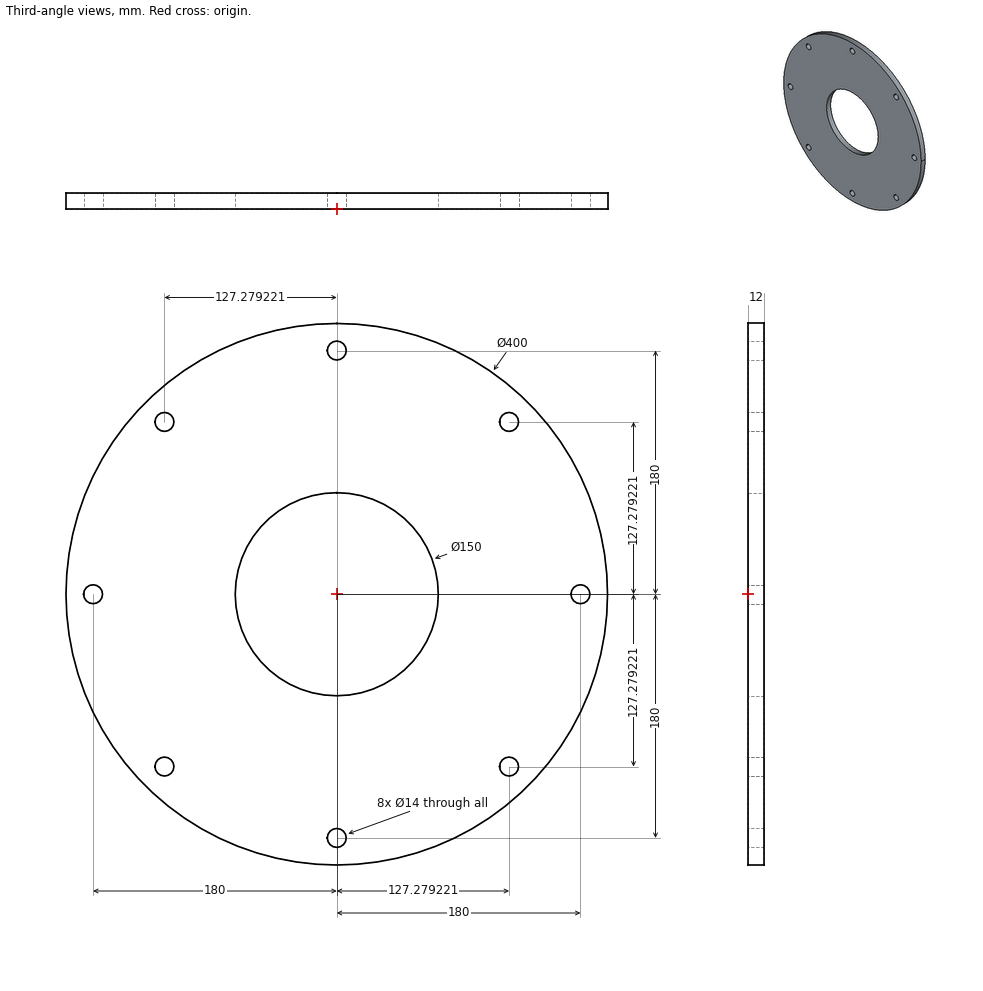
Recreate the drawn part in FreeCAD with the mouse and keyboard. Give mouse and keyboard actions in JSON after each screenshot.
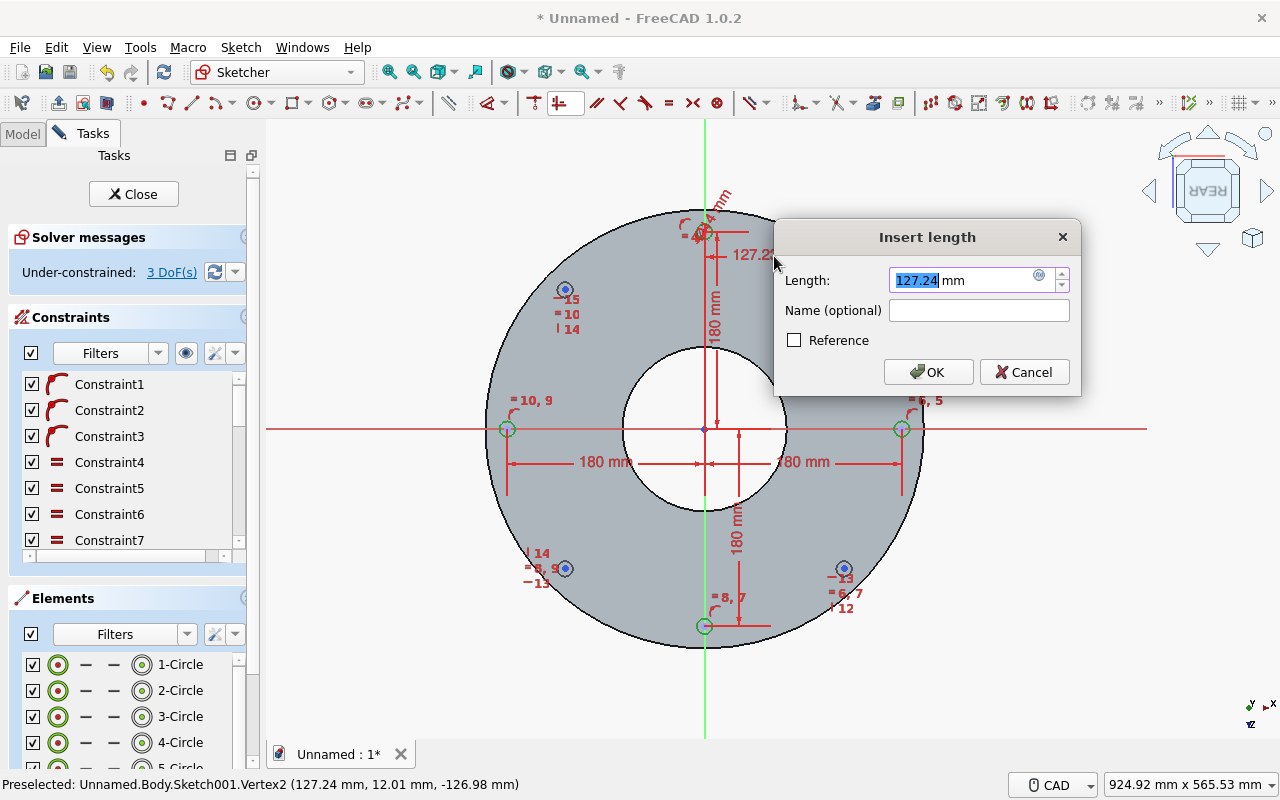
{"action": "type", "text": "127.279221"}
{"action": "key", "text": "Return"}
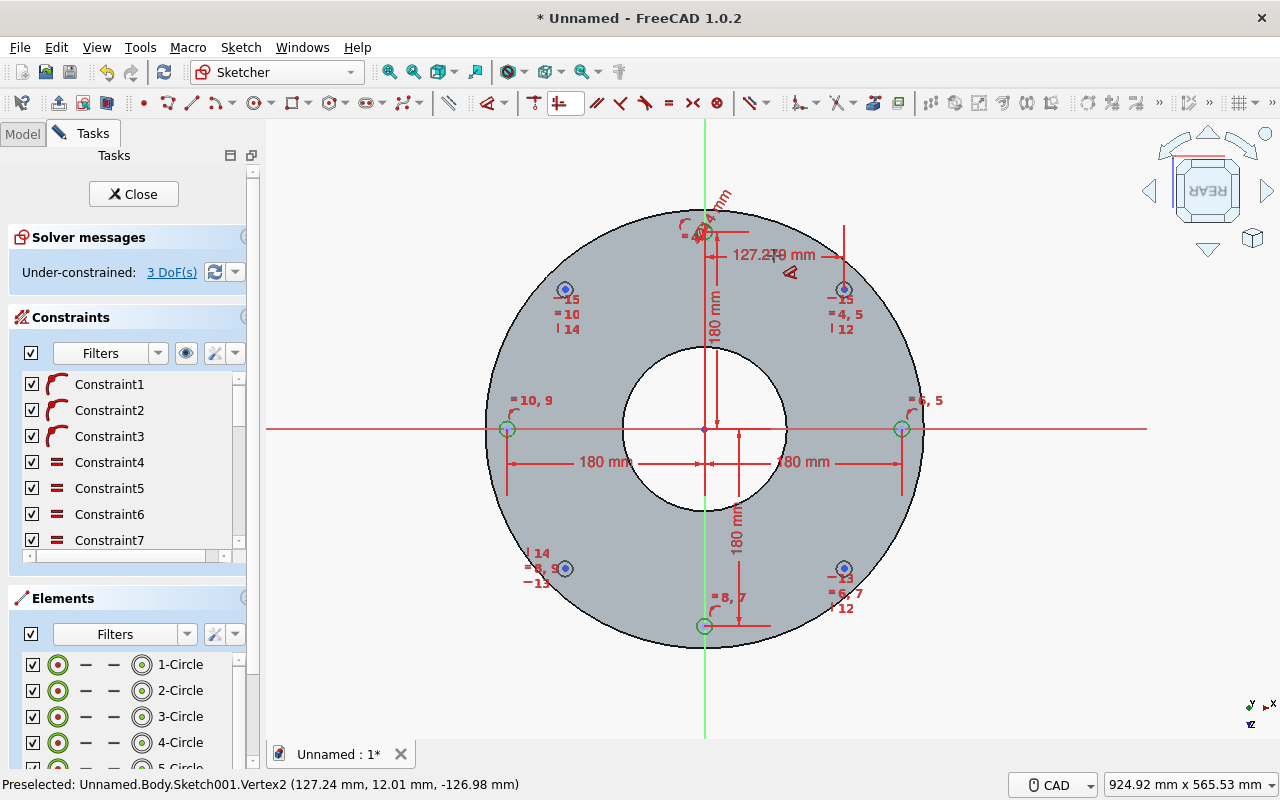
{"action": "left_click", "coordinate": [844, 290]}
{"action": "left_click", "coordinate": [878, 360]}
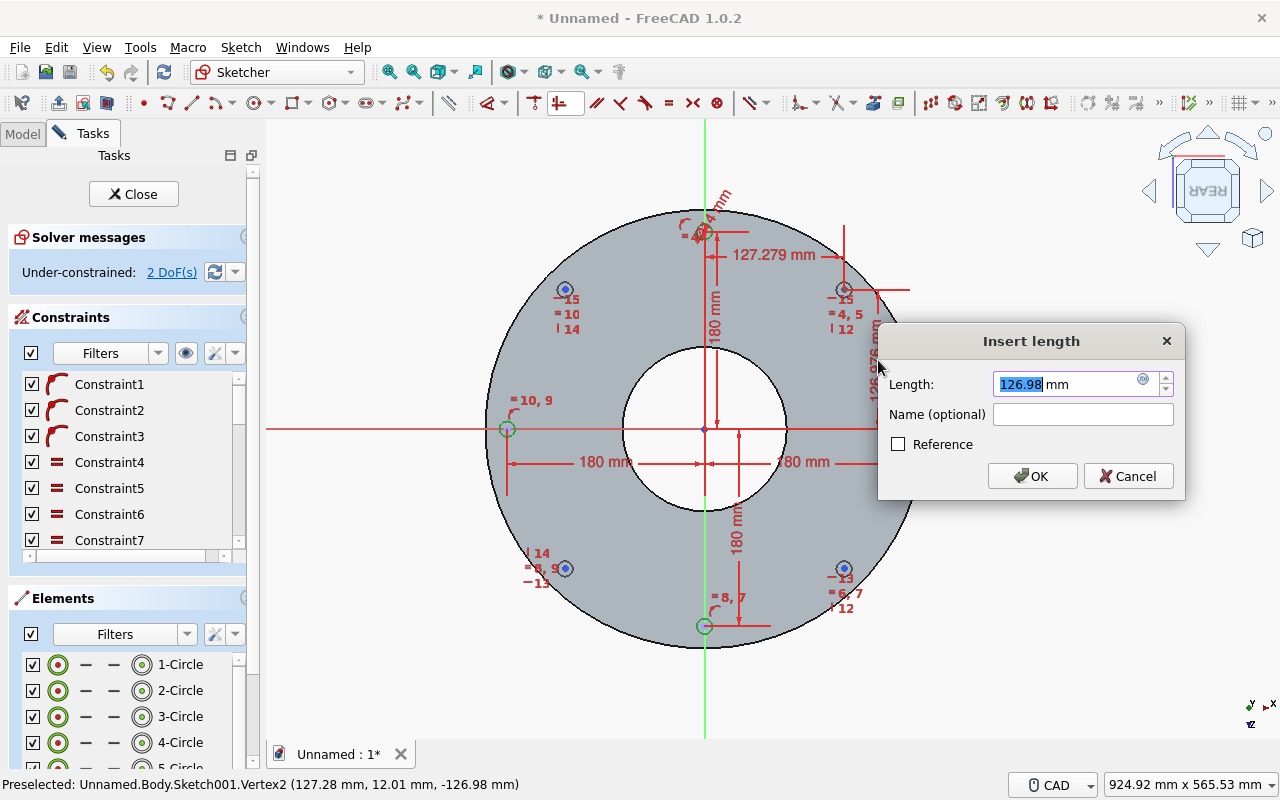
{"action": "type", "text": "127.279221"}
{"action": "key", "text": "Return"}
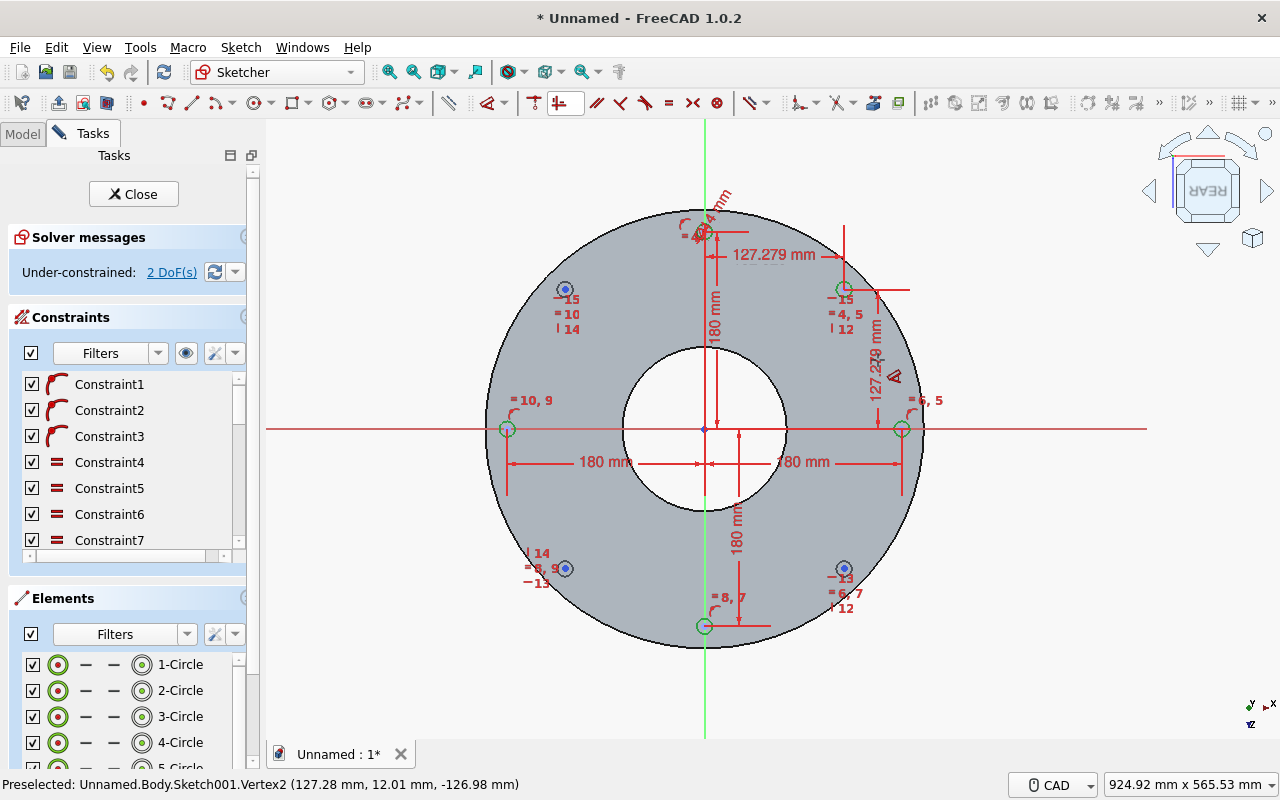
{"action": "left_click", "coordinate": [844, 569]}
{"action": "left_click", "coordinate": [878, 499]}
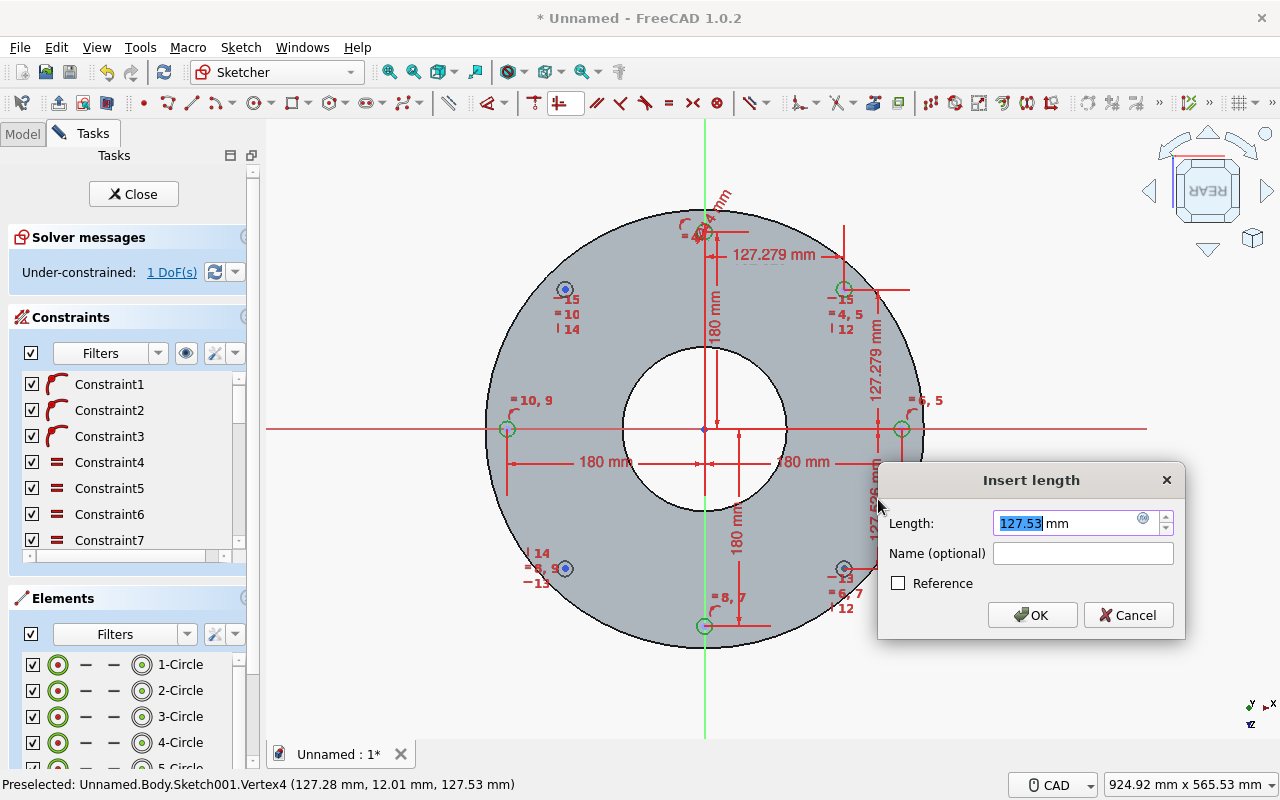
{"action": "type", "text": "127.279221"}
{"action": "key", "text": "Return"}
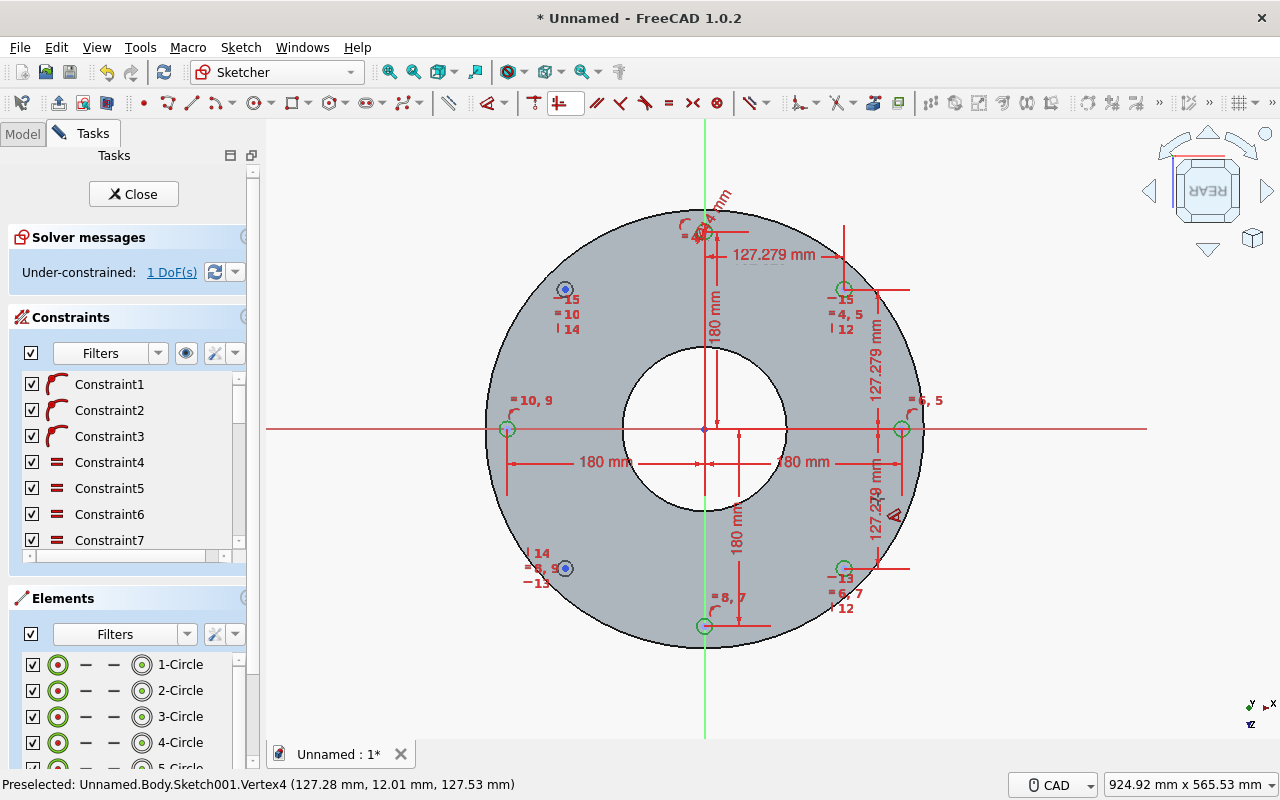
{"action": "left_click", "coordinate": [565, 569]}
{"action": "left_click", "coordinate": [635, 603]}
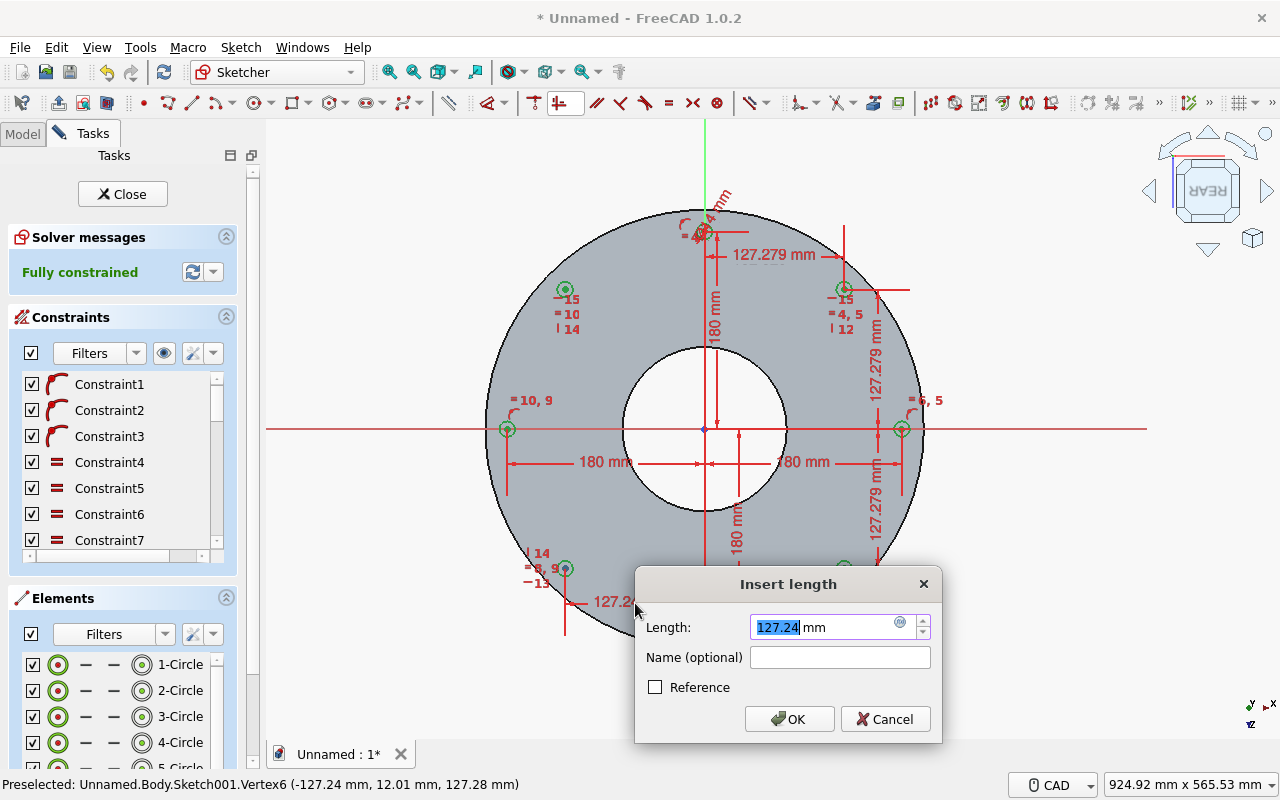
{"action": "type", "text": "127.279221"}
{"action": "key", "text": "Return"}
{"action": "key", "text": "Escape"}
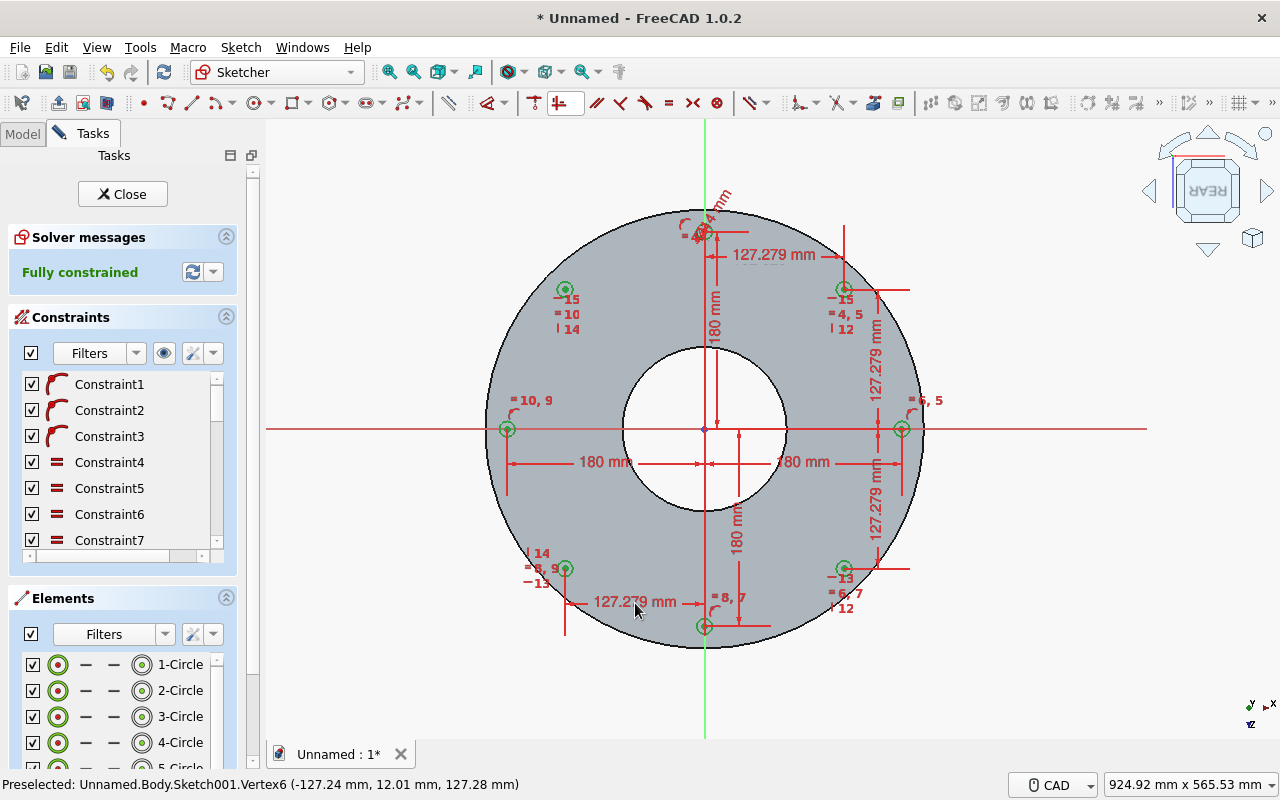
{"action": "left_click", "coordinate": [123, 194]}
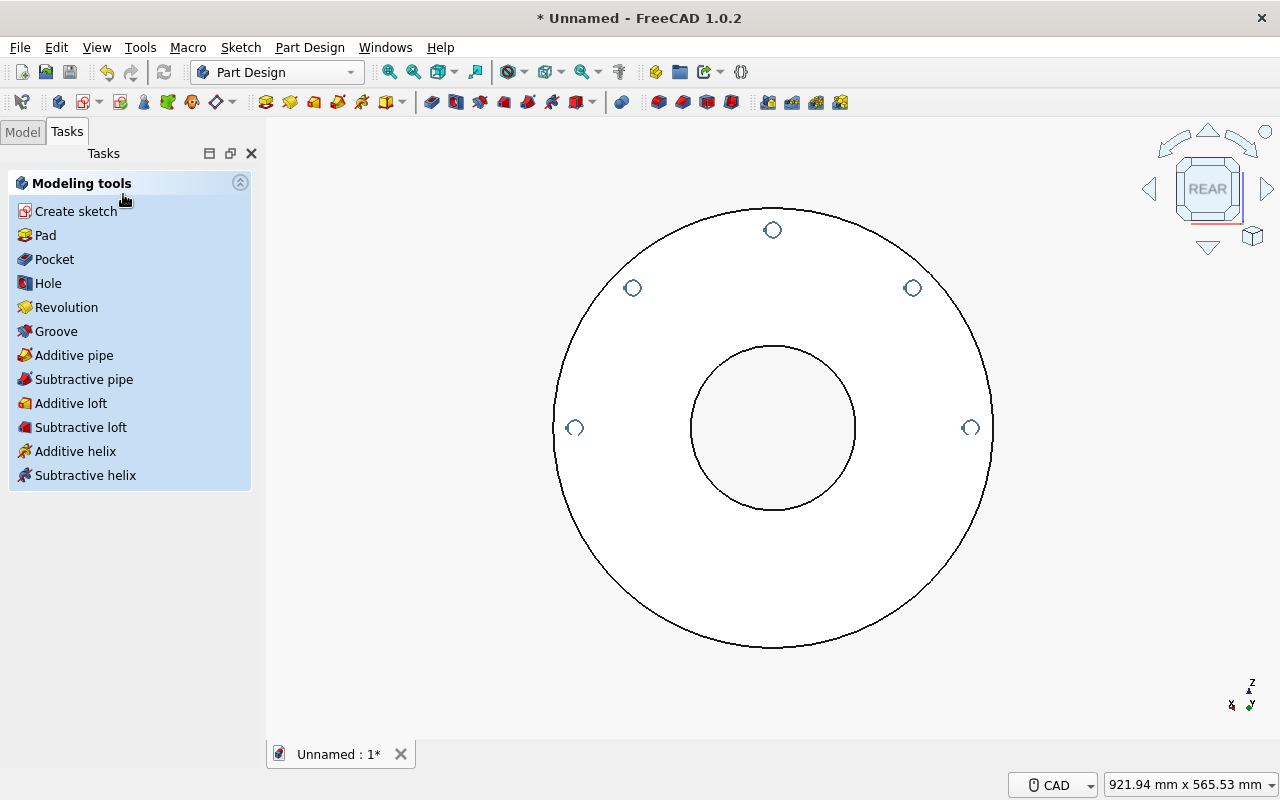
{"action": "left_click", "coordinate": [456, 102]}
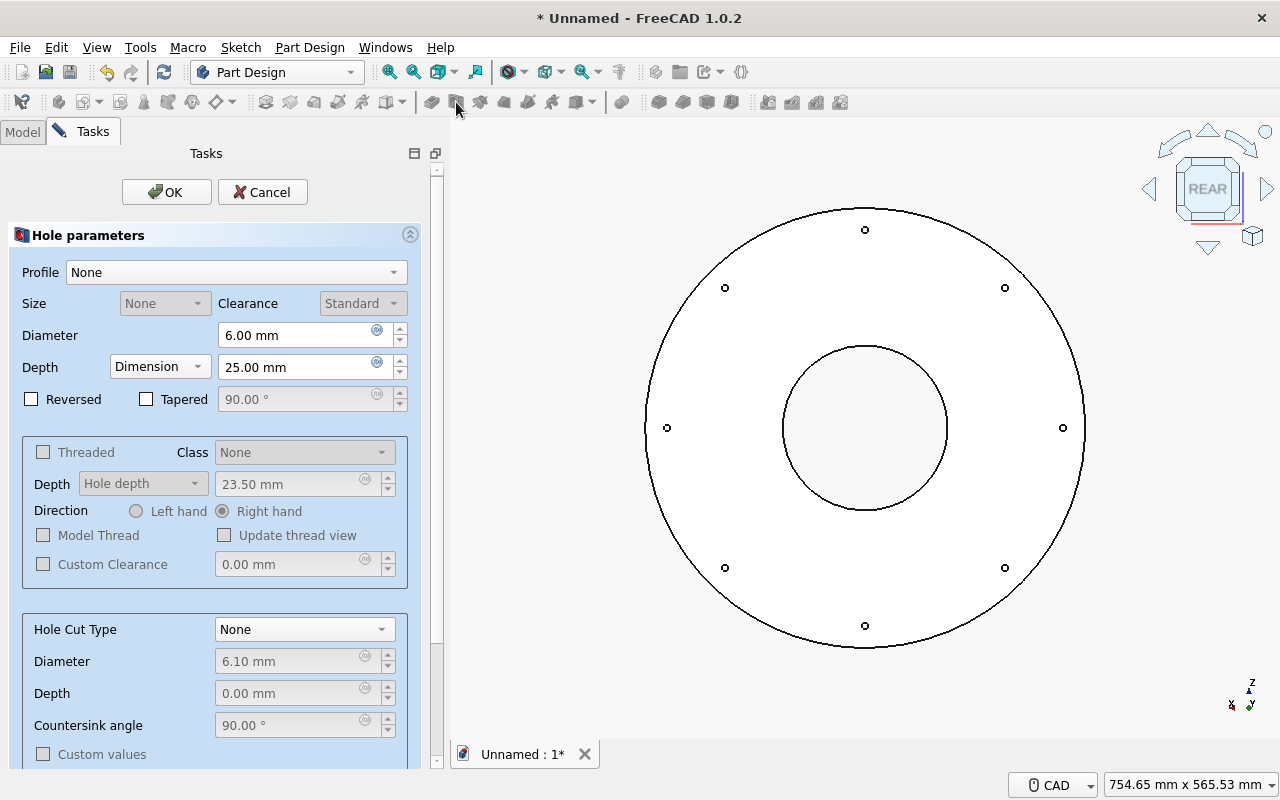
{"action": "triple_click", "coordinate": [305, 335]}